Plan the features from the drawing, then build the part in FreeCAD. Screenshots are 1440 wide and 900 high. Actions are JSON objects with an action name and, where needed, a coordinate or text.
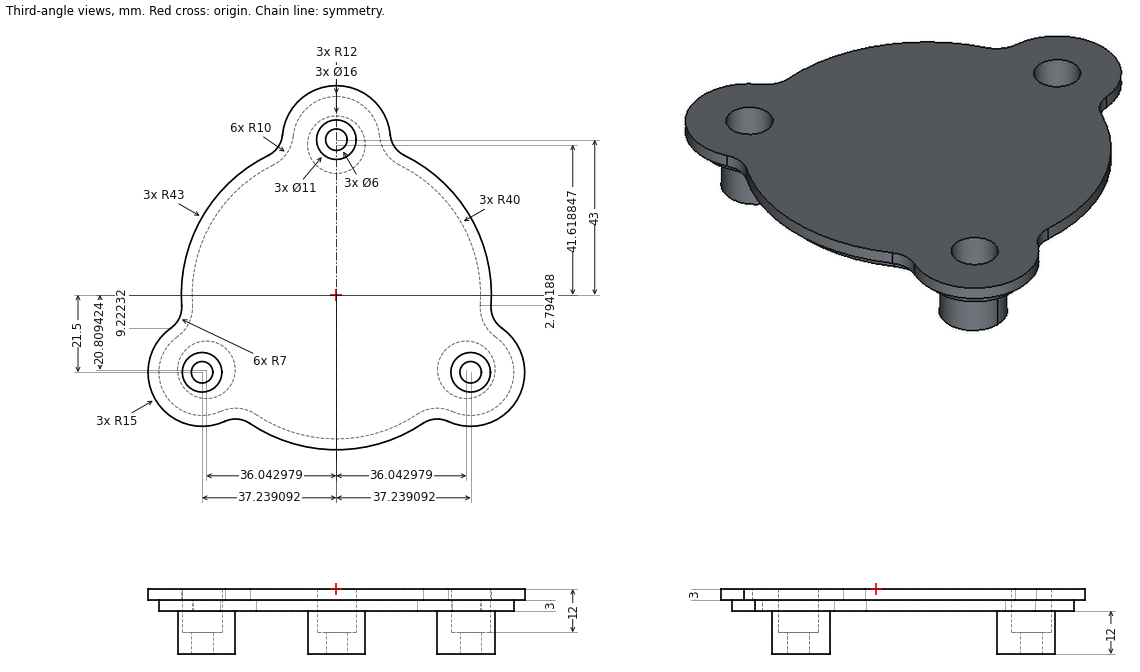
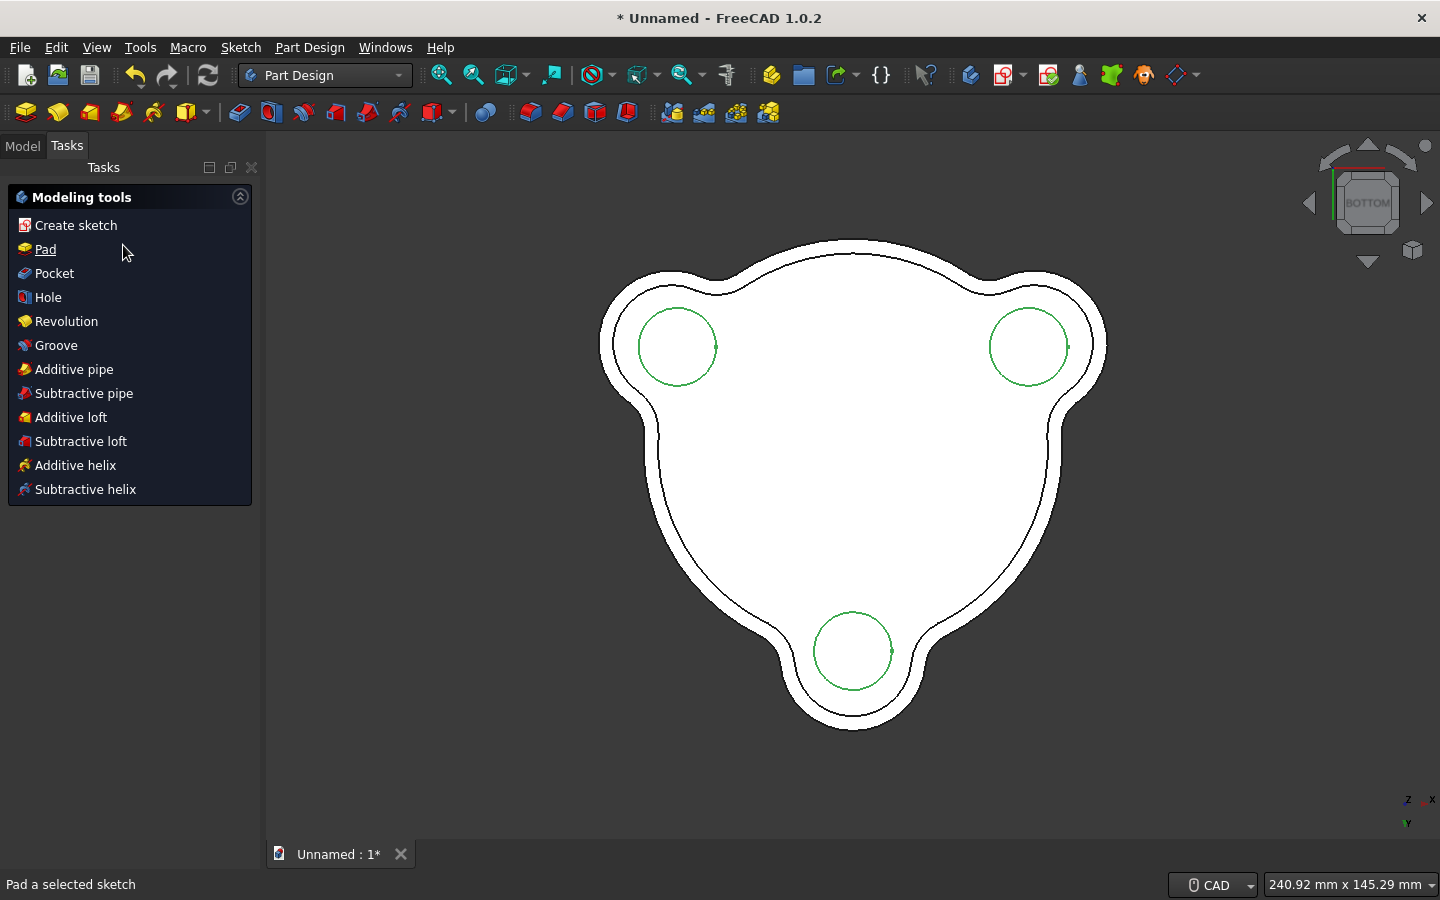
{"action": "left_click", "coordinate": [26, 112]}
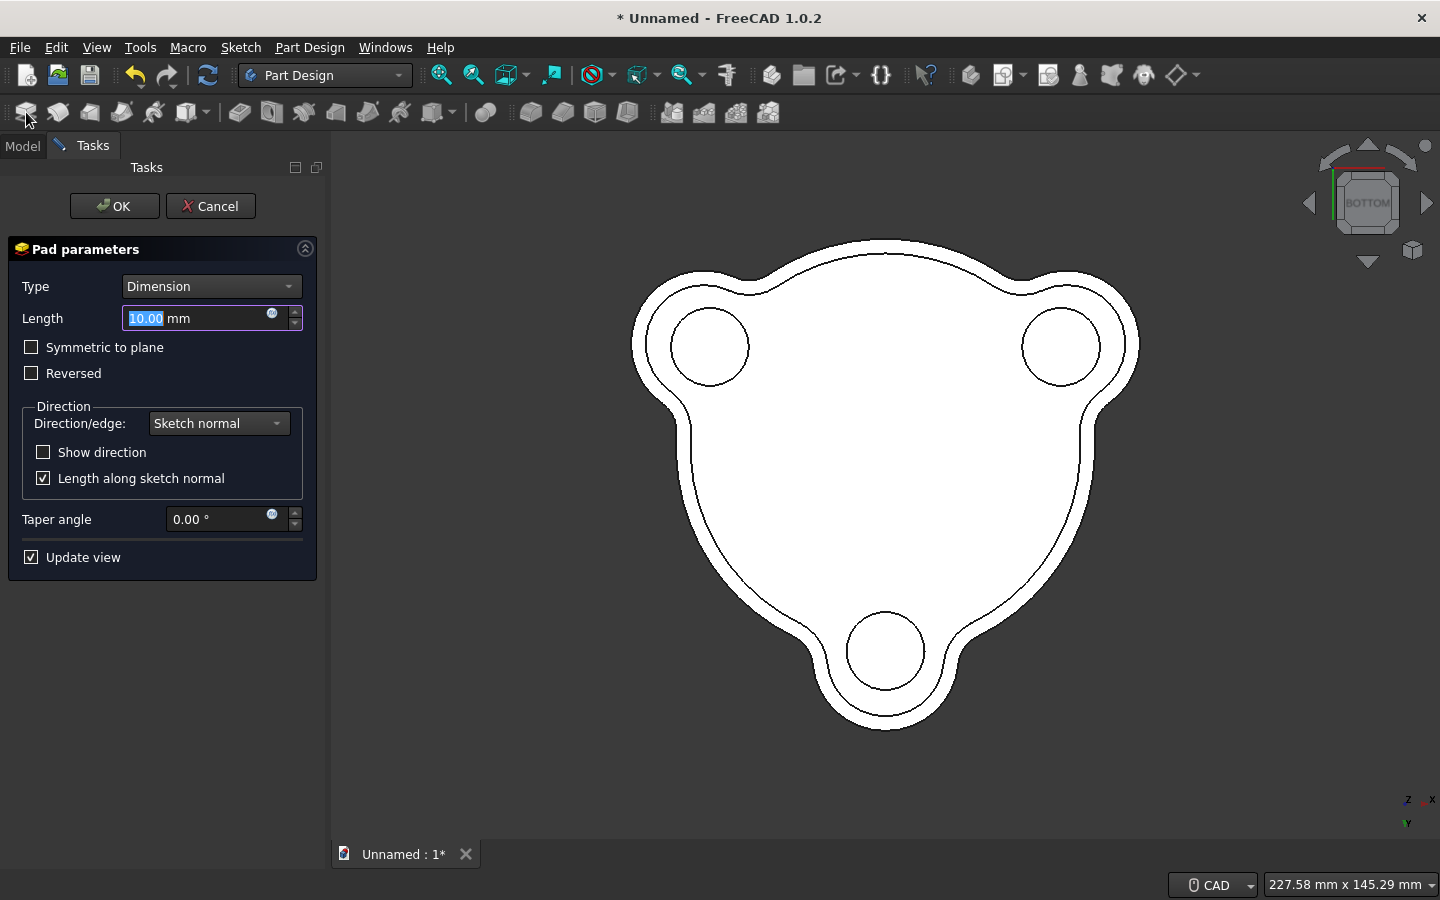
{"action": "type", "text": "12"}
{"action": "key", "text": "Tab"}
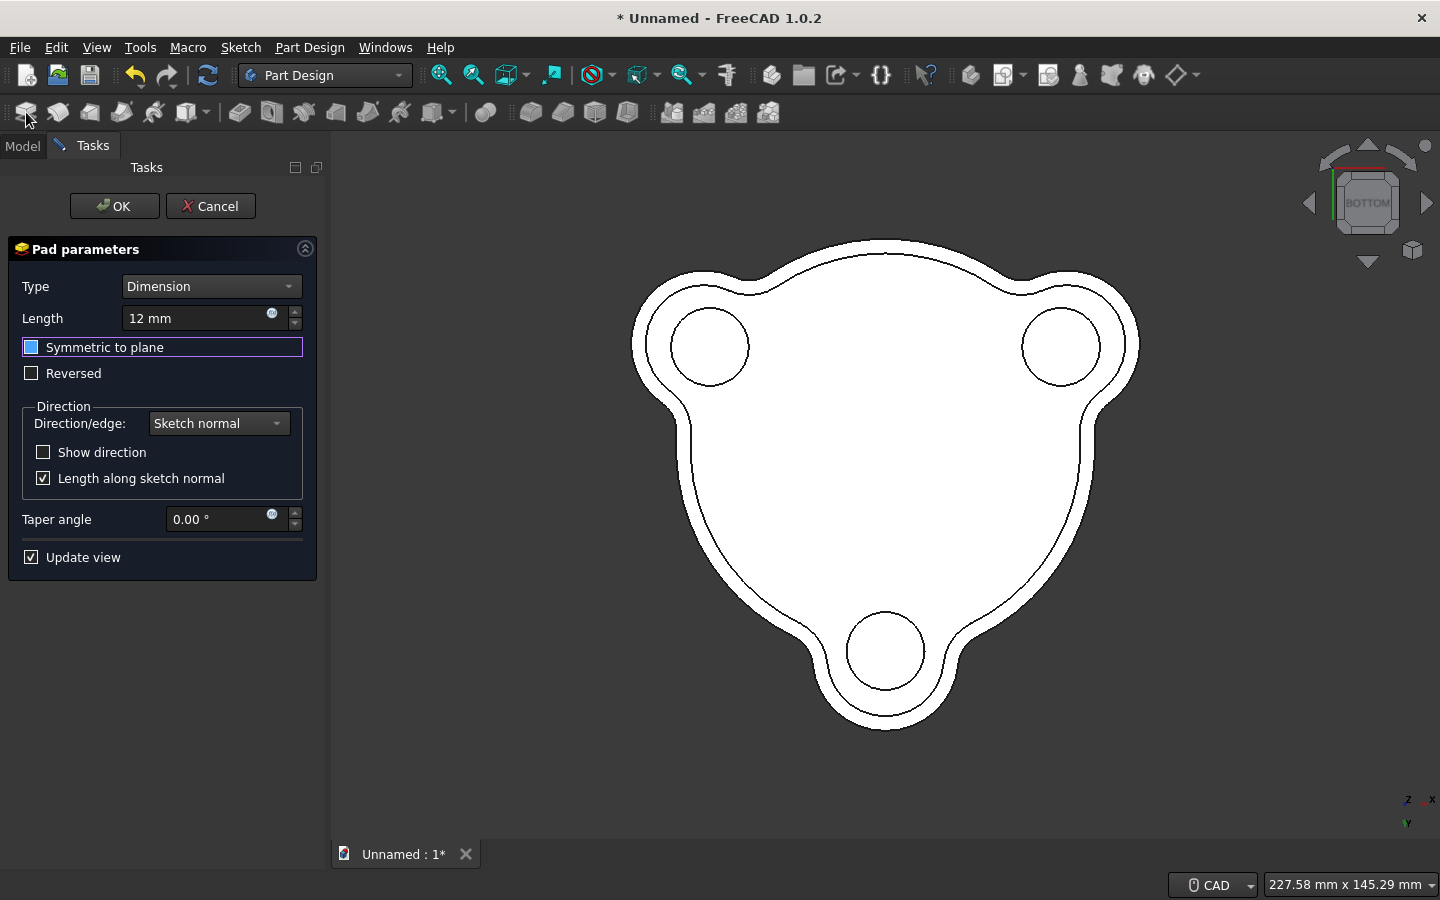
{"action": "left_click", "coordinate": [115, 206]}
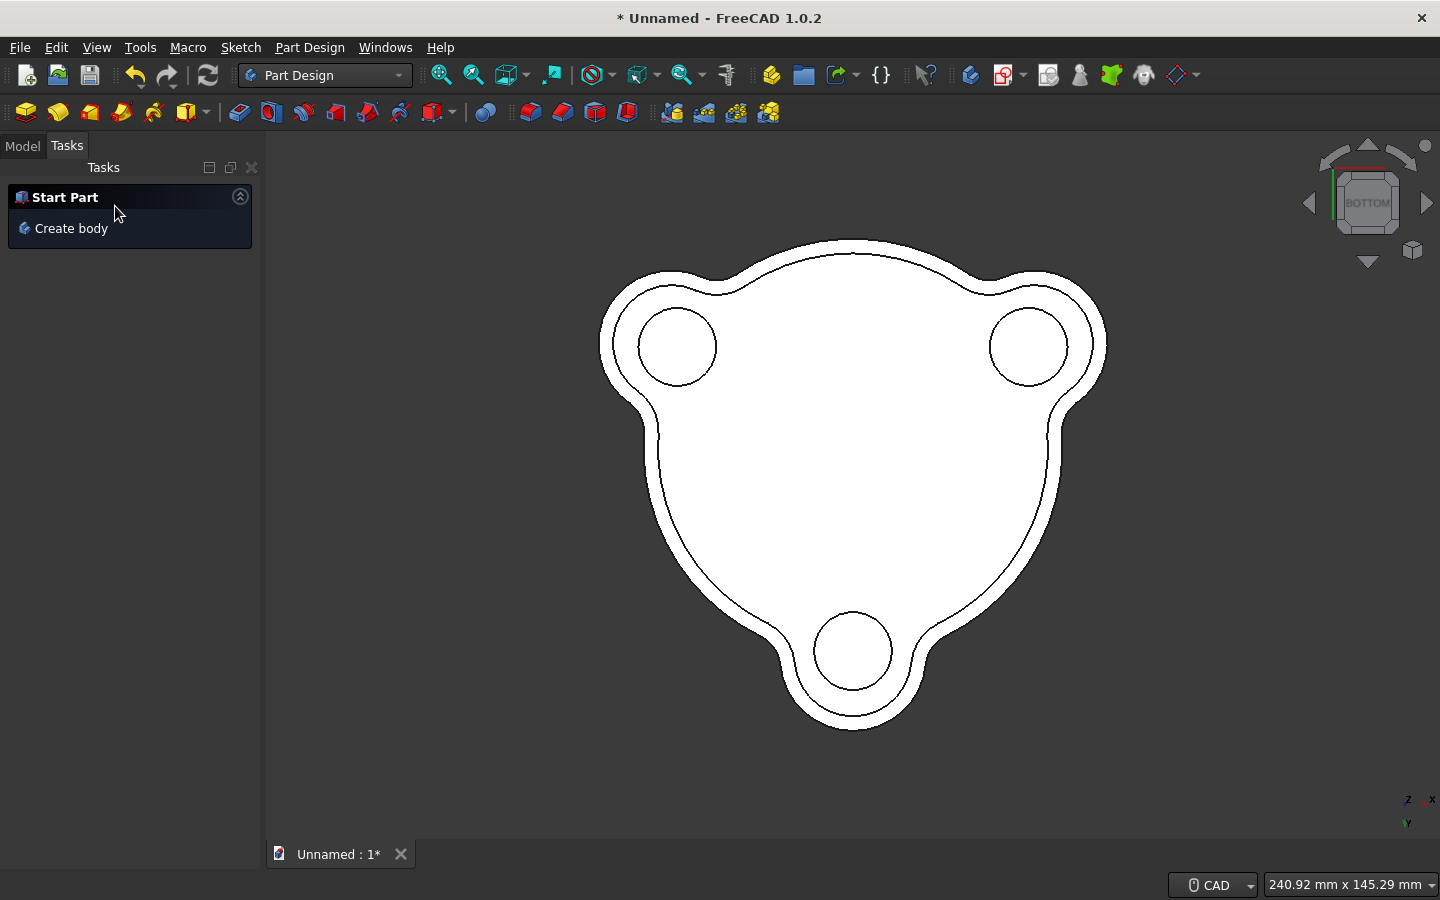
{"action": "left_click", "coordinate": [1004, 76]}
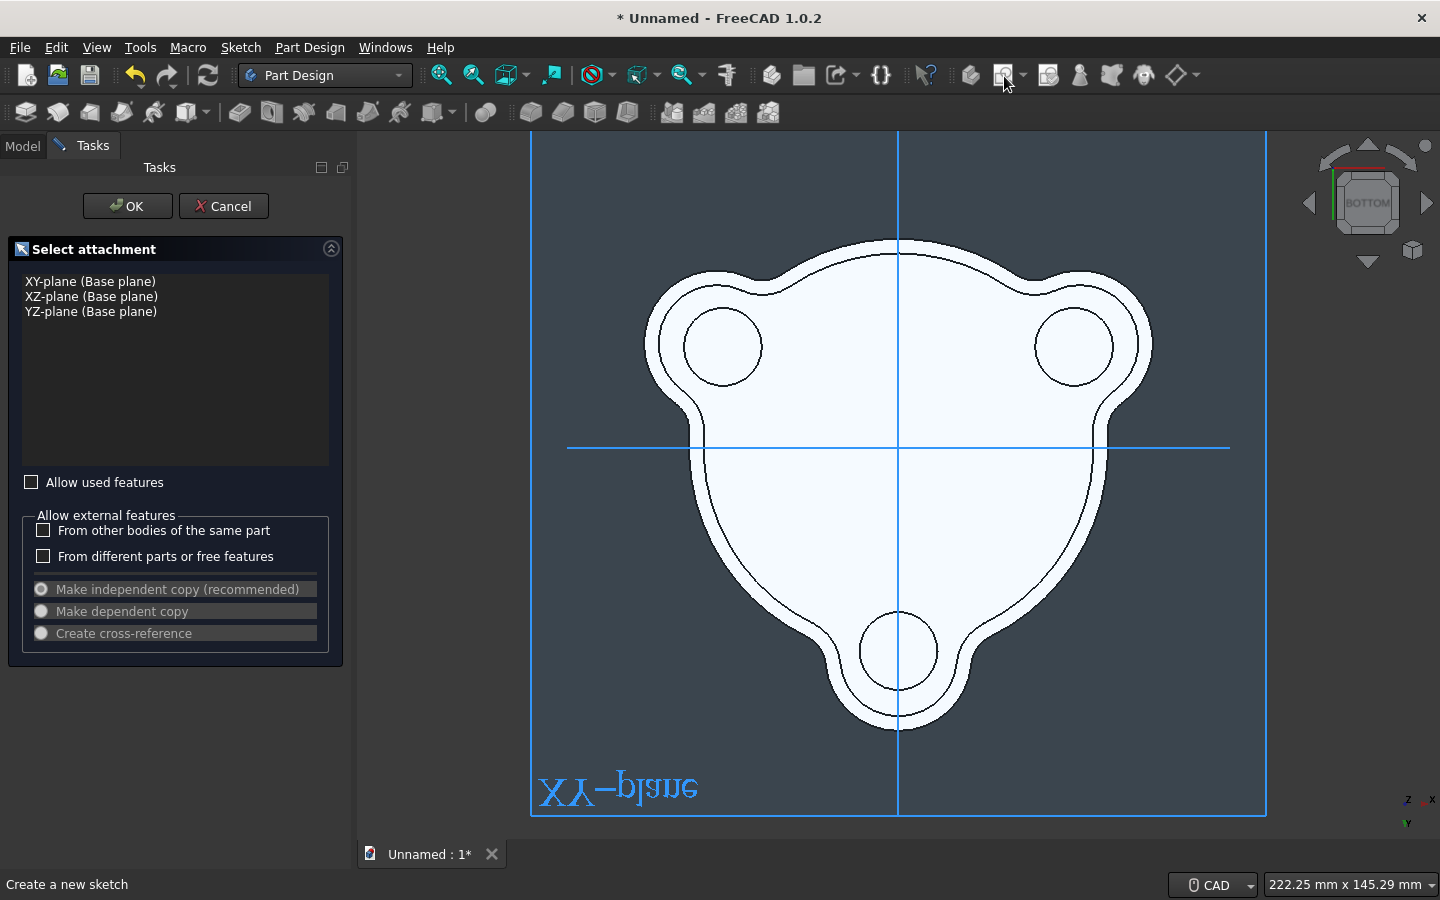
{"action": "left_click", "coordinate": [82, 282]}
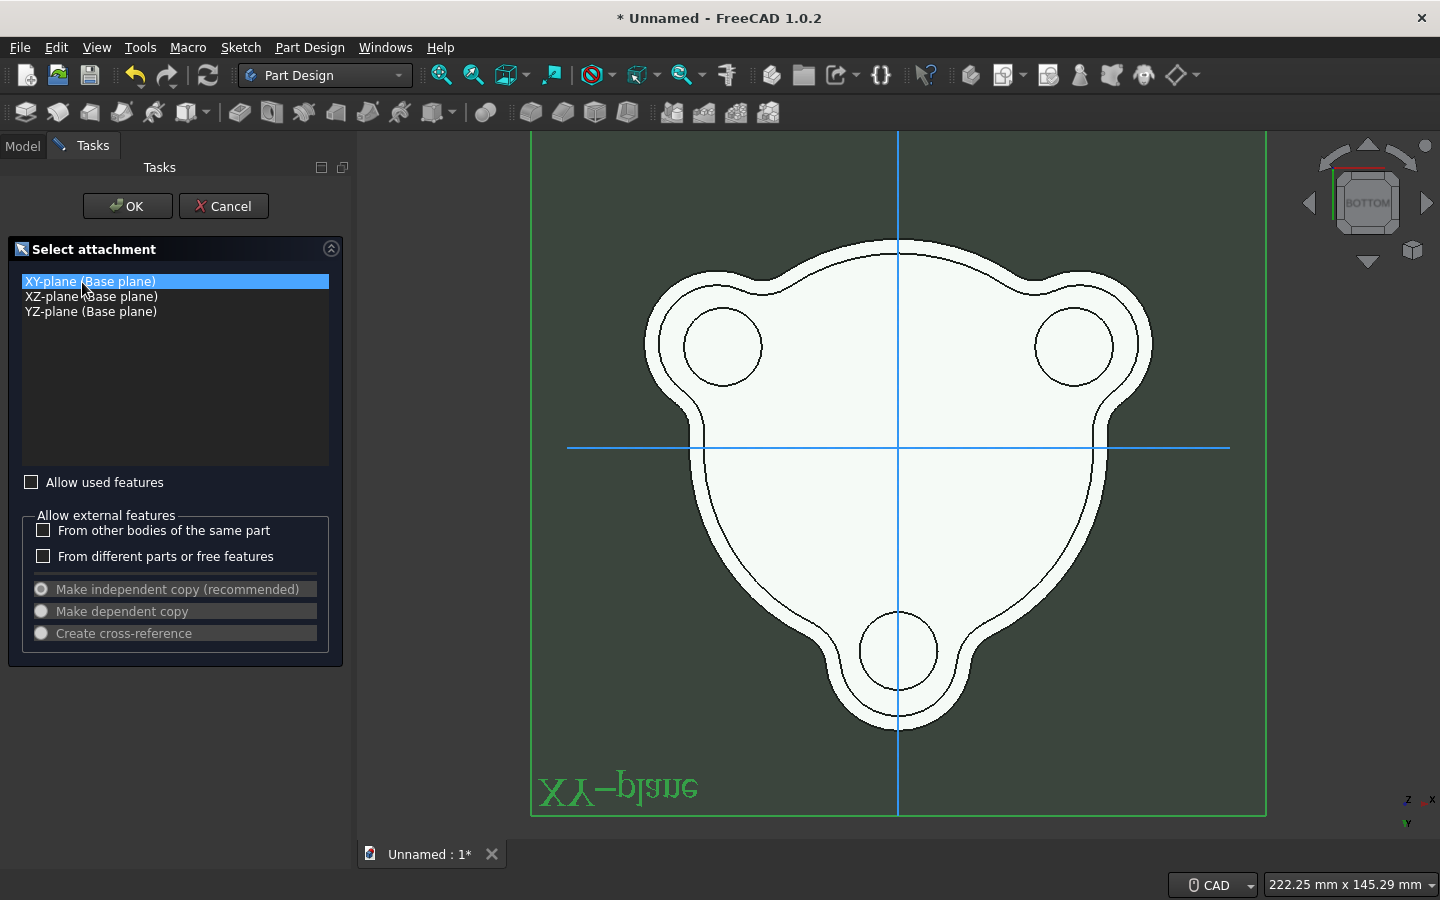
{"action": "left_click", "coordinate": [128, 206]}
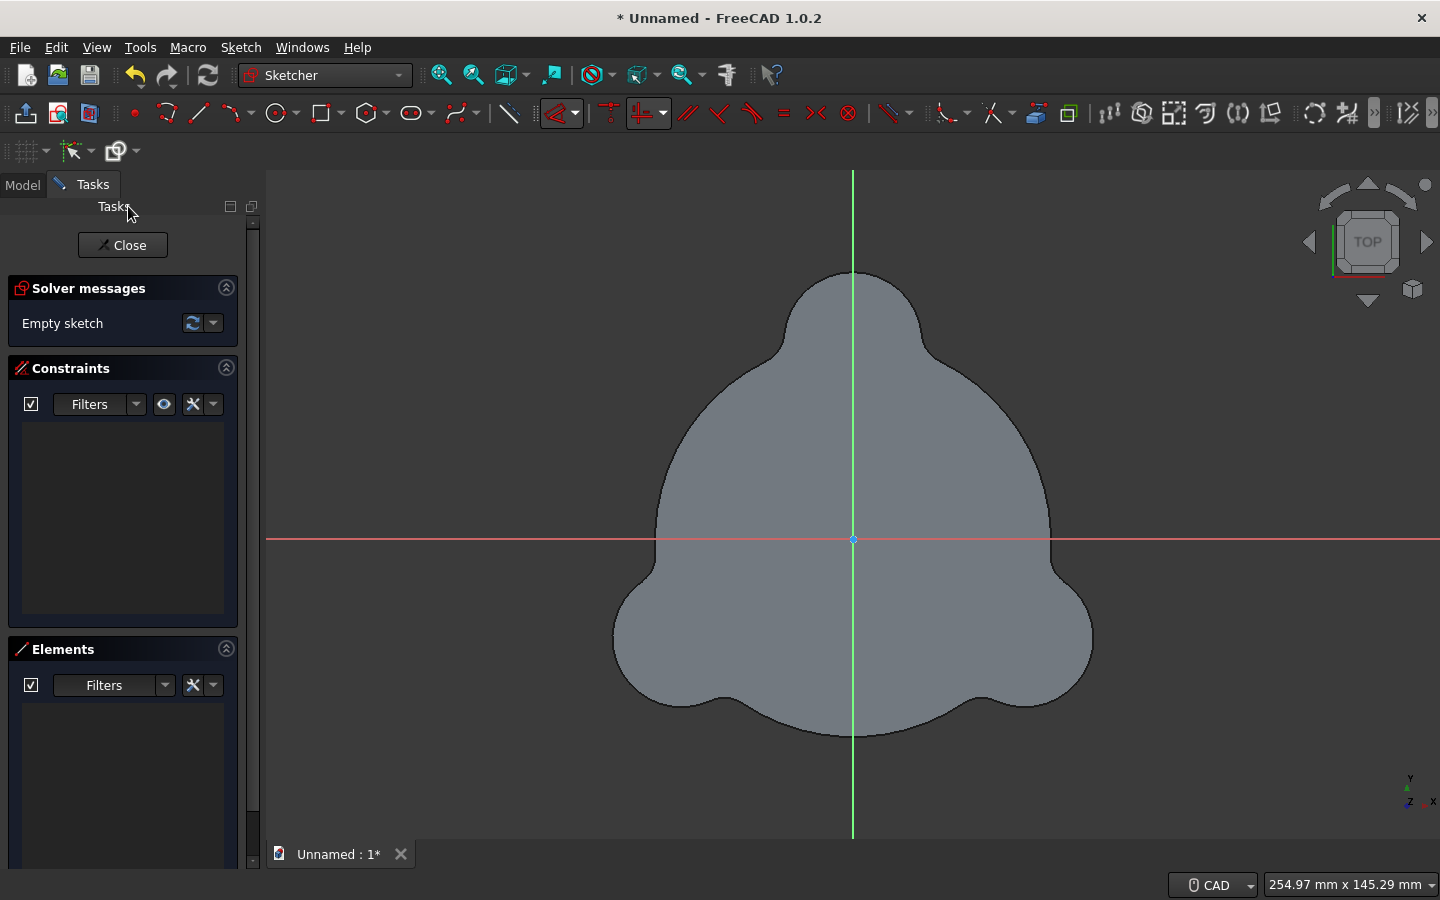
{"action": "left_click", "coordinate": [276, 114]}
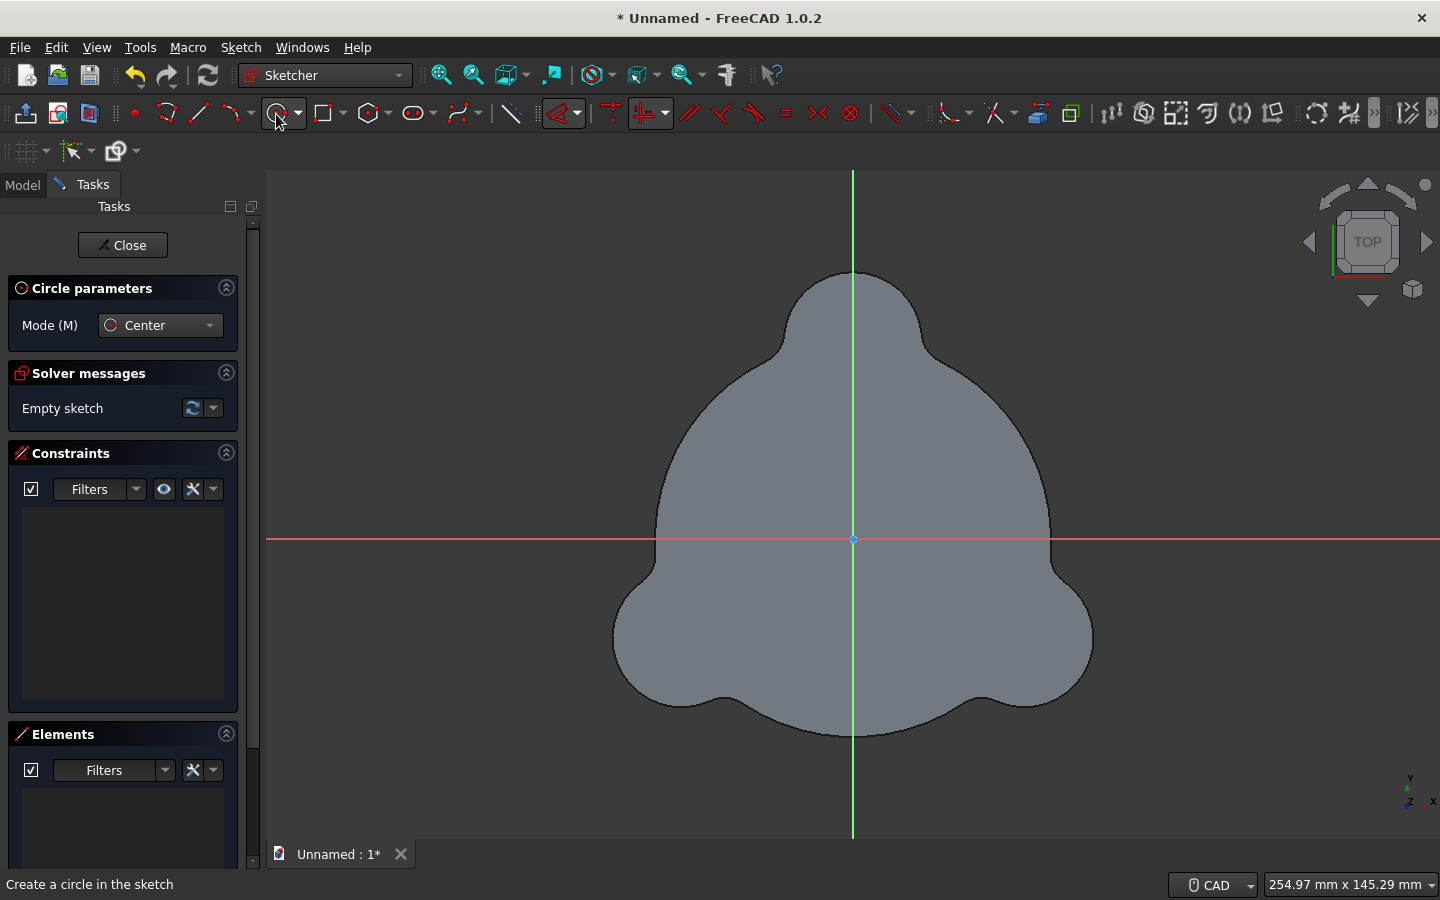
{"action": "left_click", "coordinate": [853, 341]}
{"action": "left_click", "coordinate": [871, 323]}